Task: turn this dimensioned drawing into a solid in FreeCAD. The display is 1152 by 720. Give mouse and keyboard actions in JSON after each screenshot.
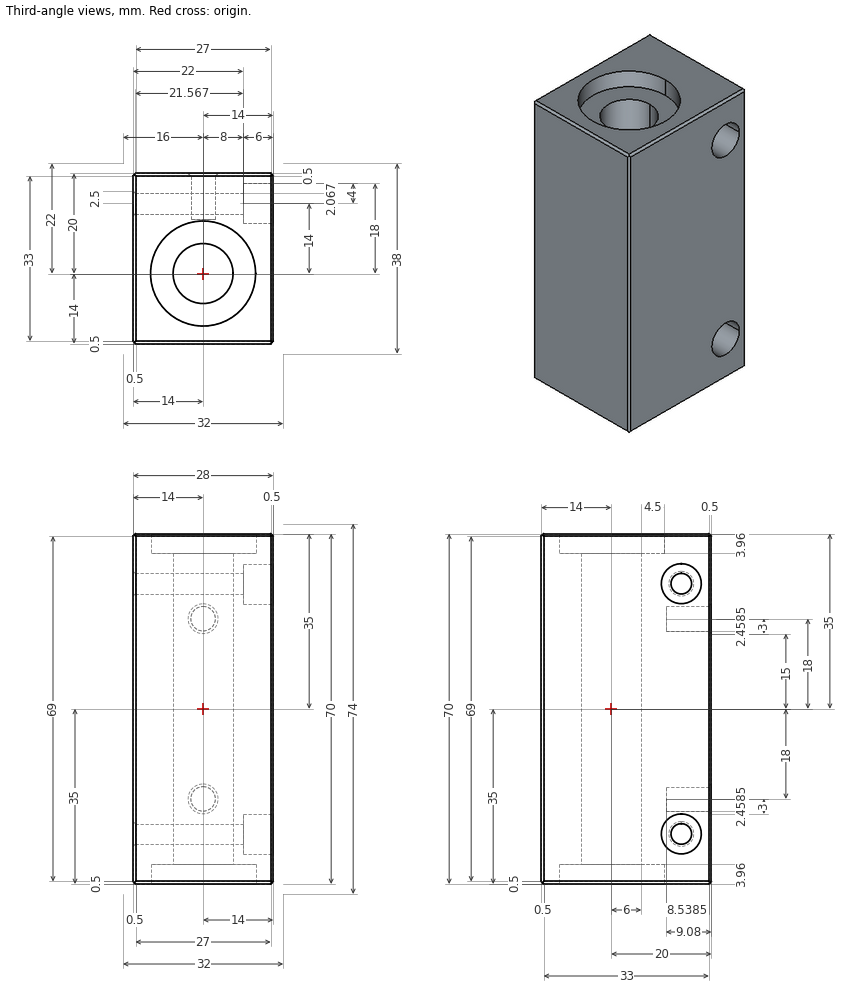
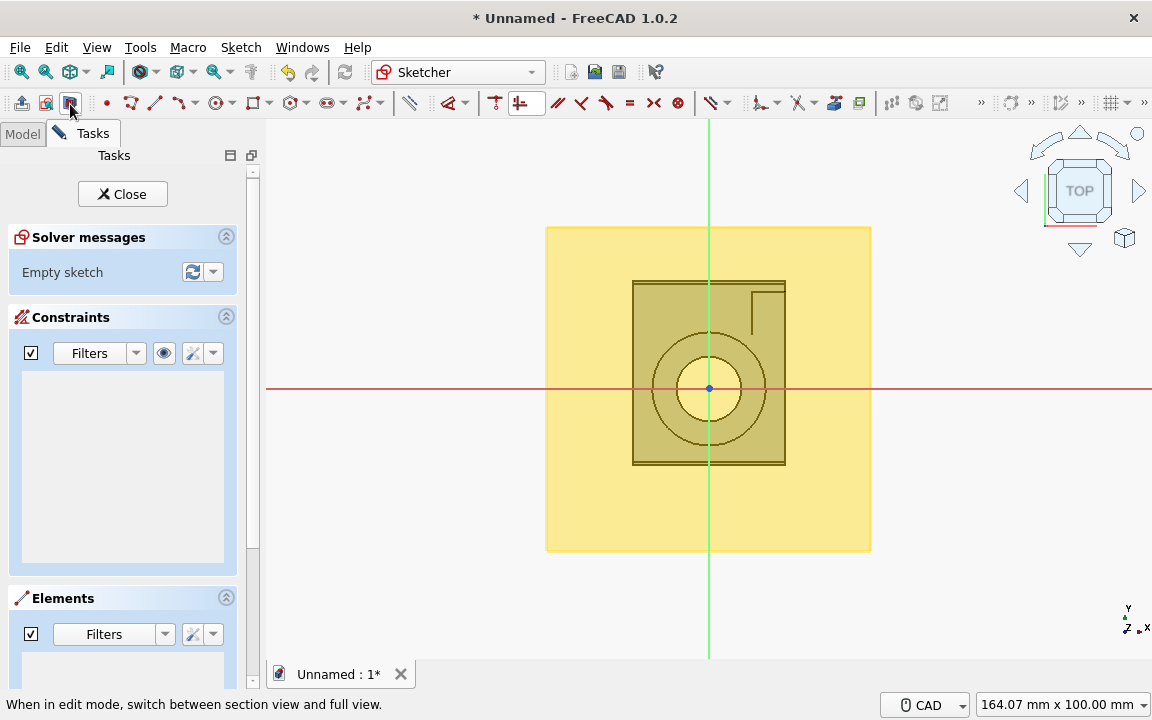
{"action": "scroll", "coordinate": [686, 319], "scroll_direction": "up", "scroll_amount": 5}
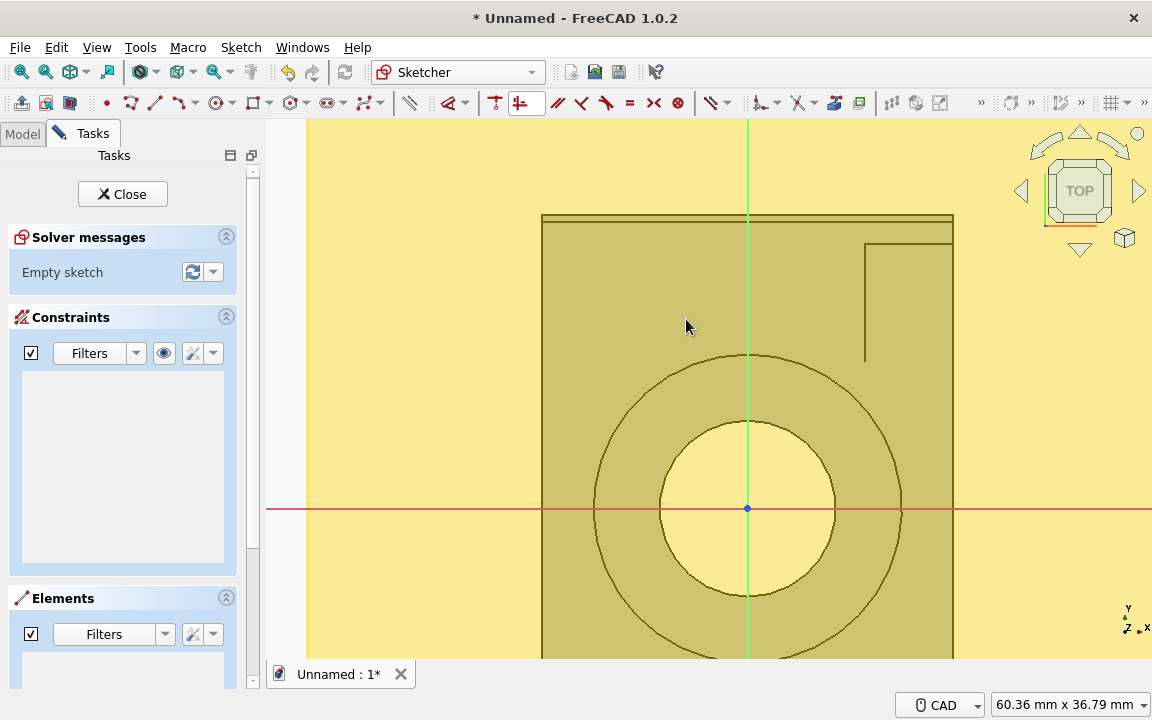
{"action": "left_click", "coordinate": [132, 104]}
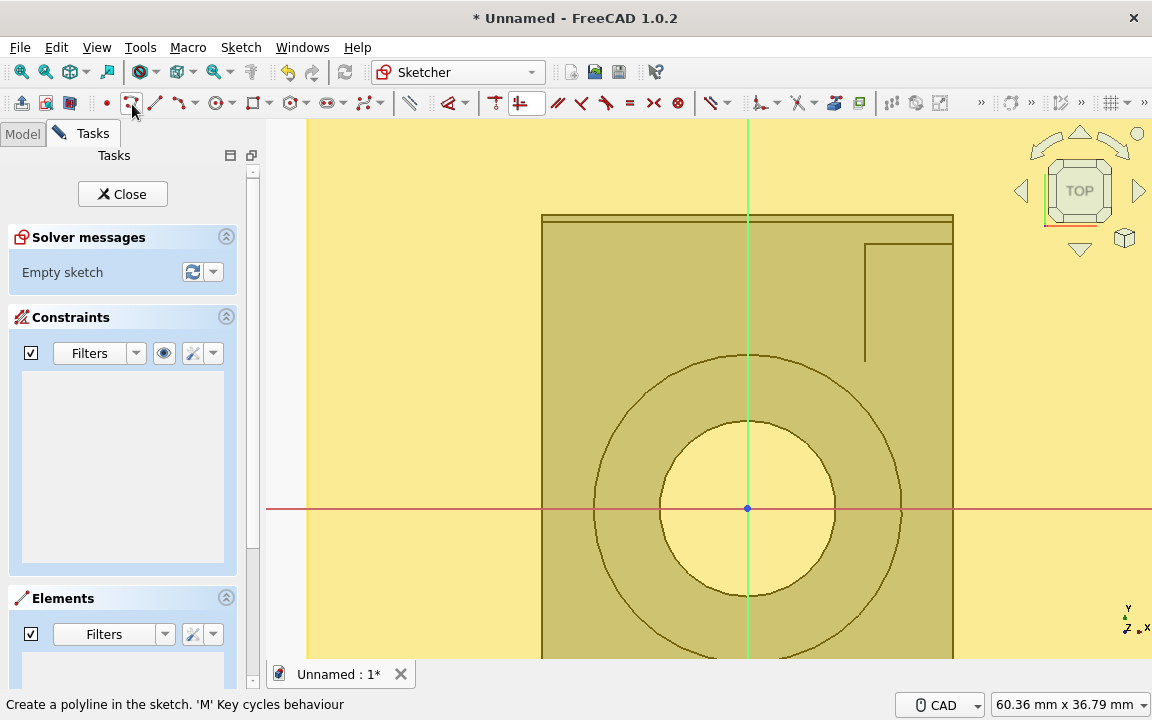
{"action": "left_click", "coordinate": [865, 303]}
{"action": "left_click", "coordinate": [865, 273]}
{"action": "left_click", "coordinate": [549, 273]}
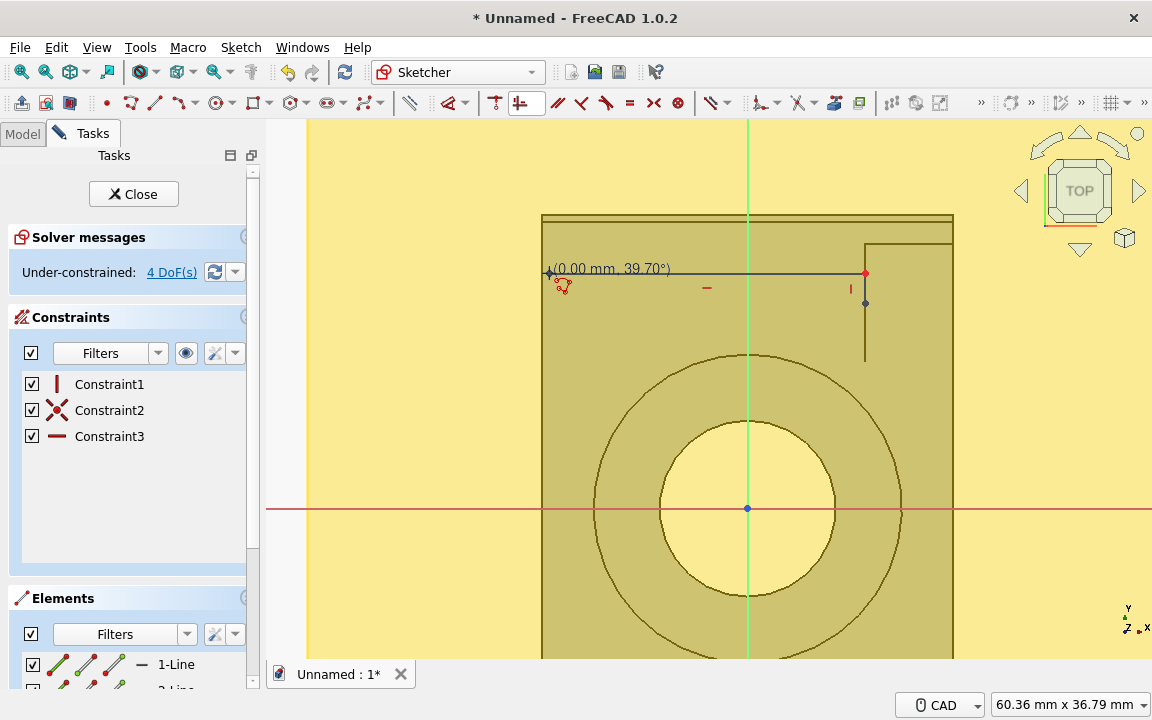
{"action": "scroll", "coordinate": [542, 266], "scroll_direction": "up", "scroll_amount": 3}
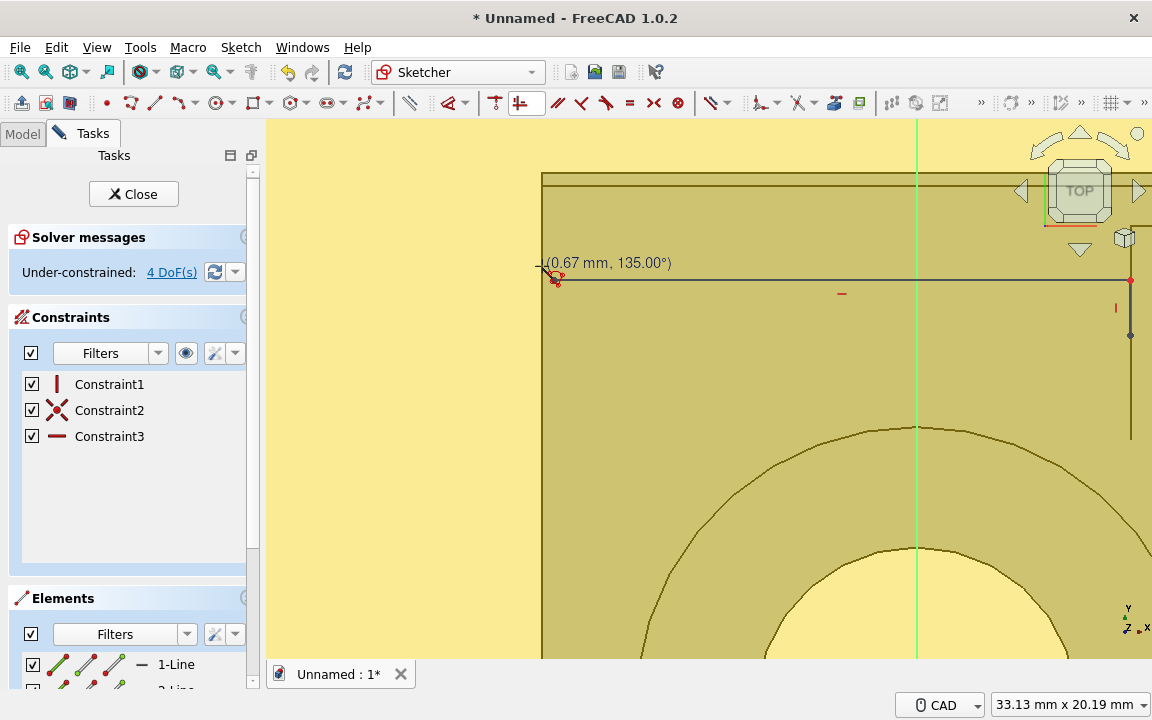
{"action": "left_click", "coordinate": [542, 267]}
{"action": "left_click", "coordinate": [542, 333]}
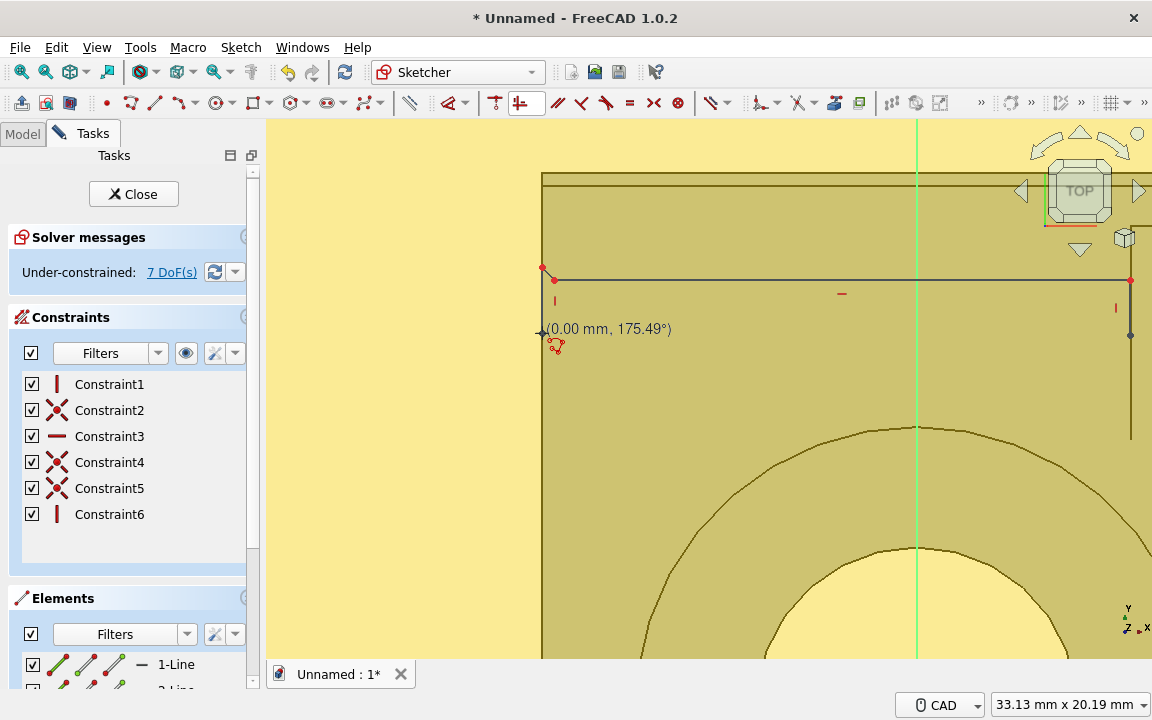
{"action": "scroll", "coordinate": [545, 270], "scroll_direction": "down", "scroll_amount": 3}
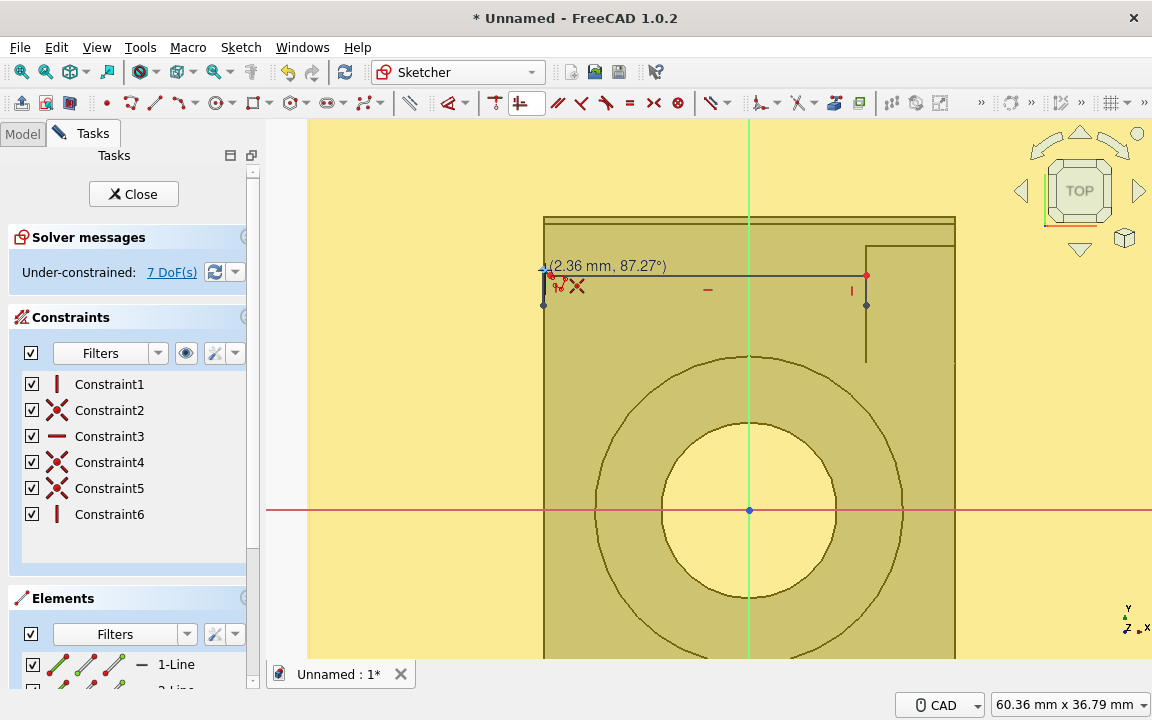
{"action": "left_click", "coordinate": [866, 306]}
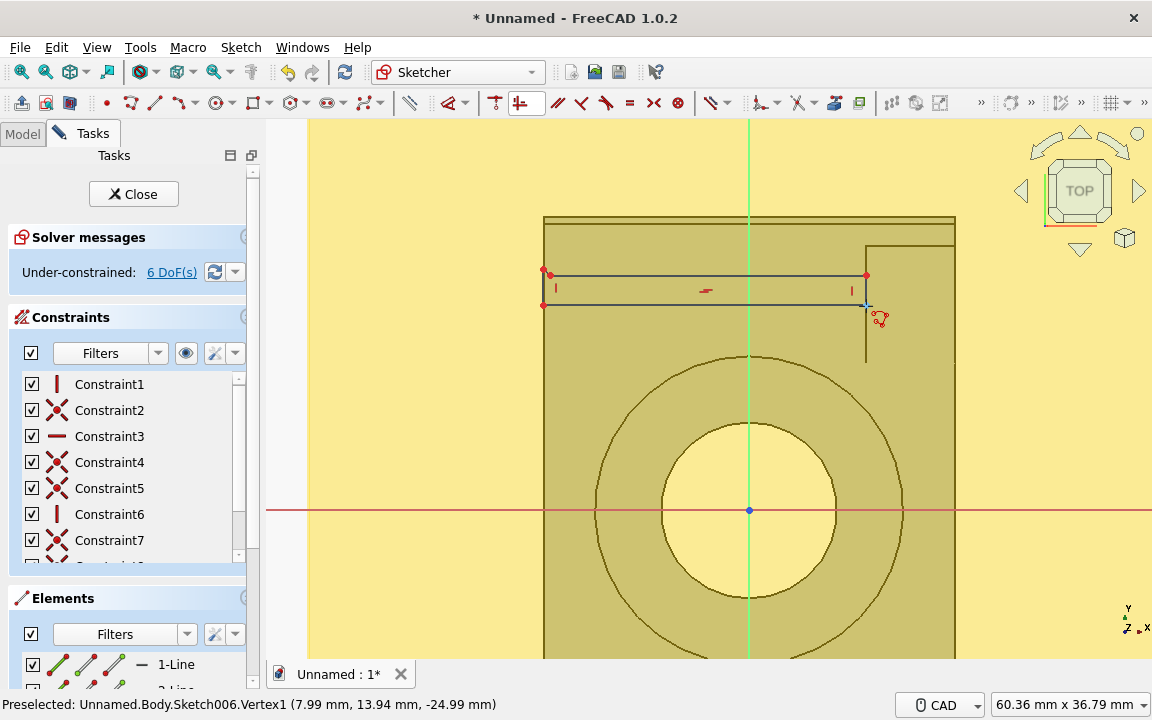
{"action": "left_click", "coordinate": [156, 104]}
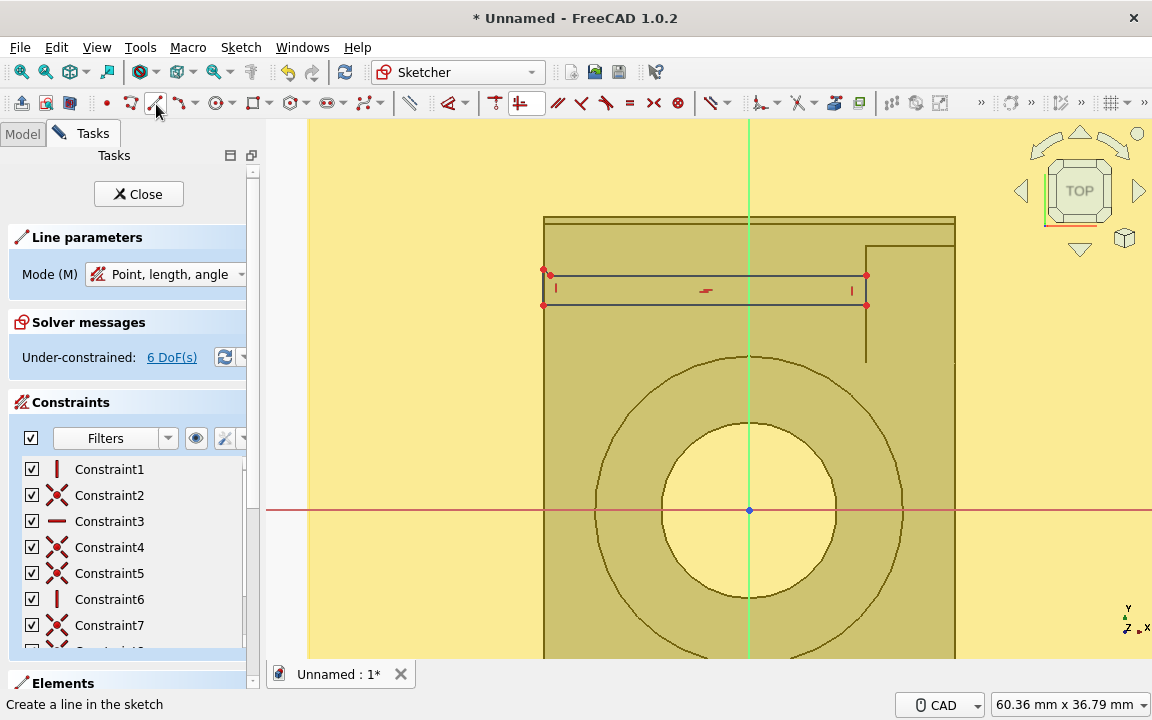
{"action": "left_click", "coordinate": [511, 305]}
{"action": "left_click", "coordinate": [414, 305]}
{"action": "key", "text": "Escape"}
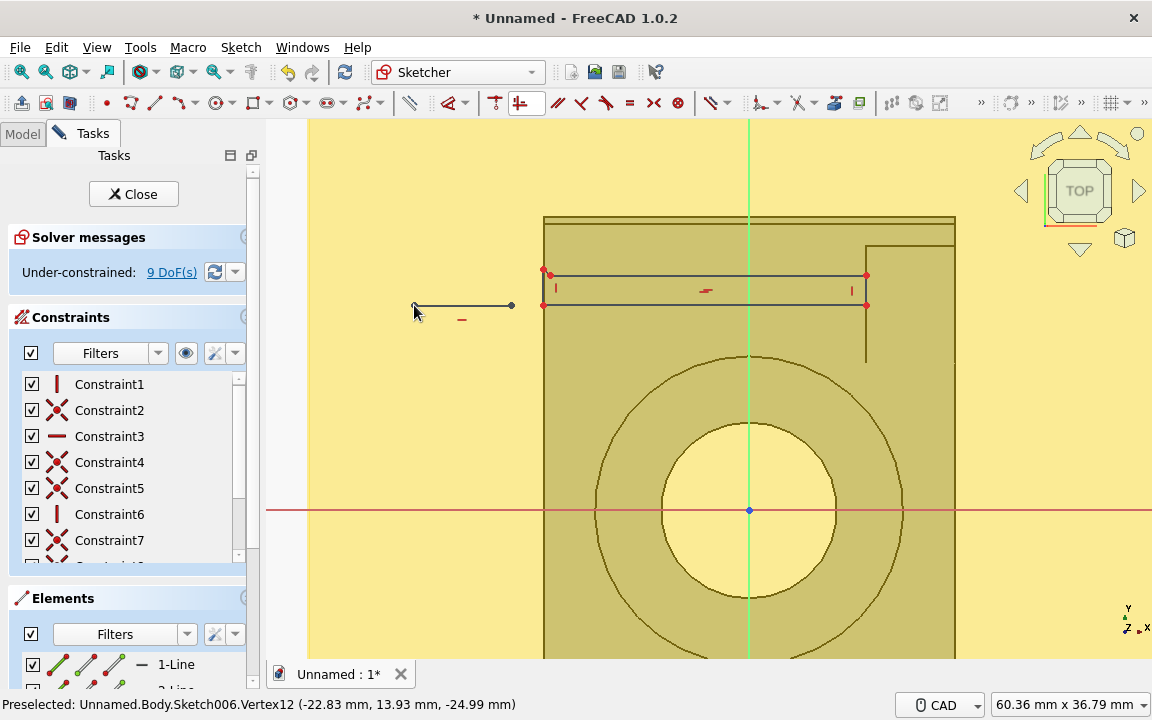
{"action": "left_click", "coordinate": [482, 306]}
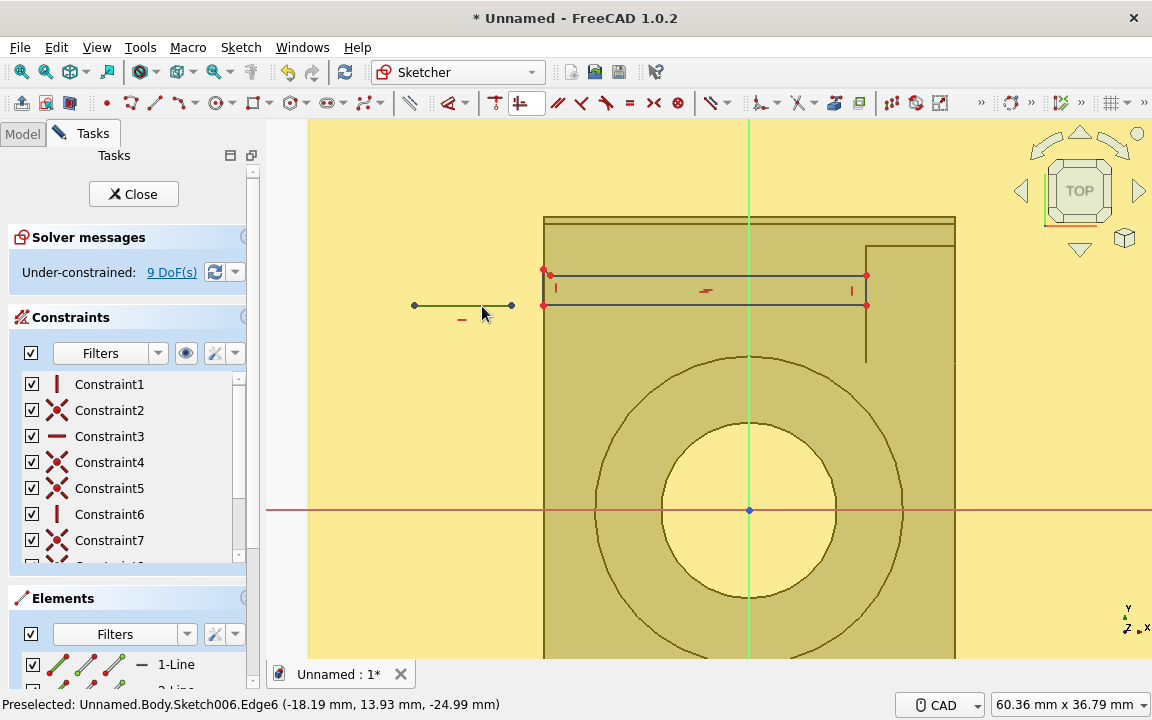
{"action": "left_click", "coordinate": [410, 104]}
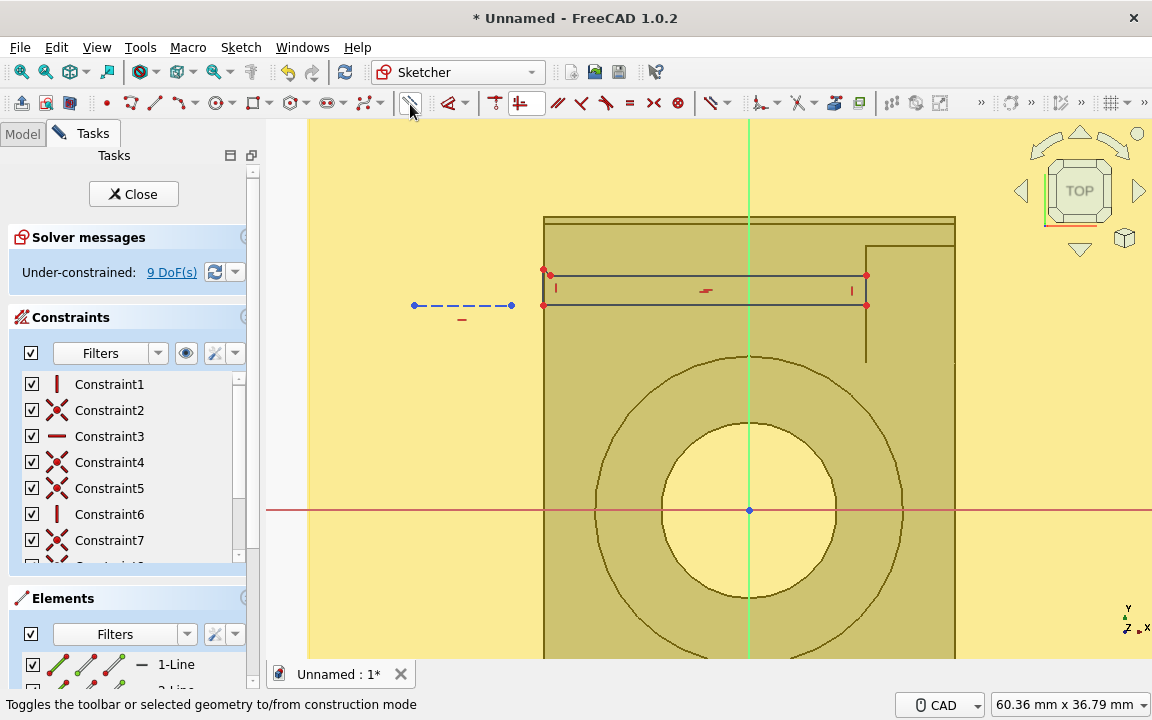
{"action": "left_click", "coordinate": [448, 104]}